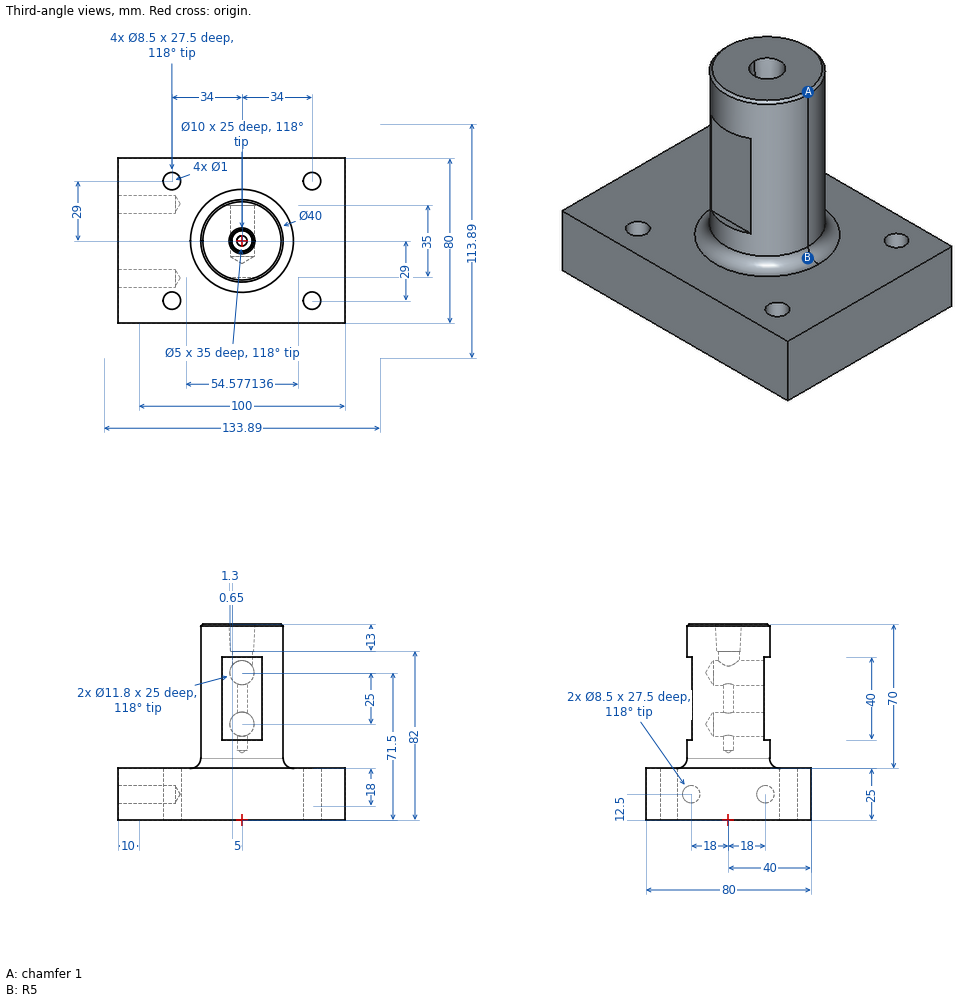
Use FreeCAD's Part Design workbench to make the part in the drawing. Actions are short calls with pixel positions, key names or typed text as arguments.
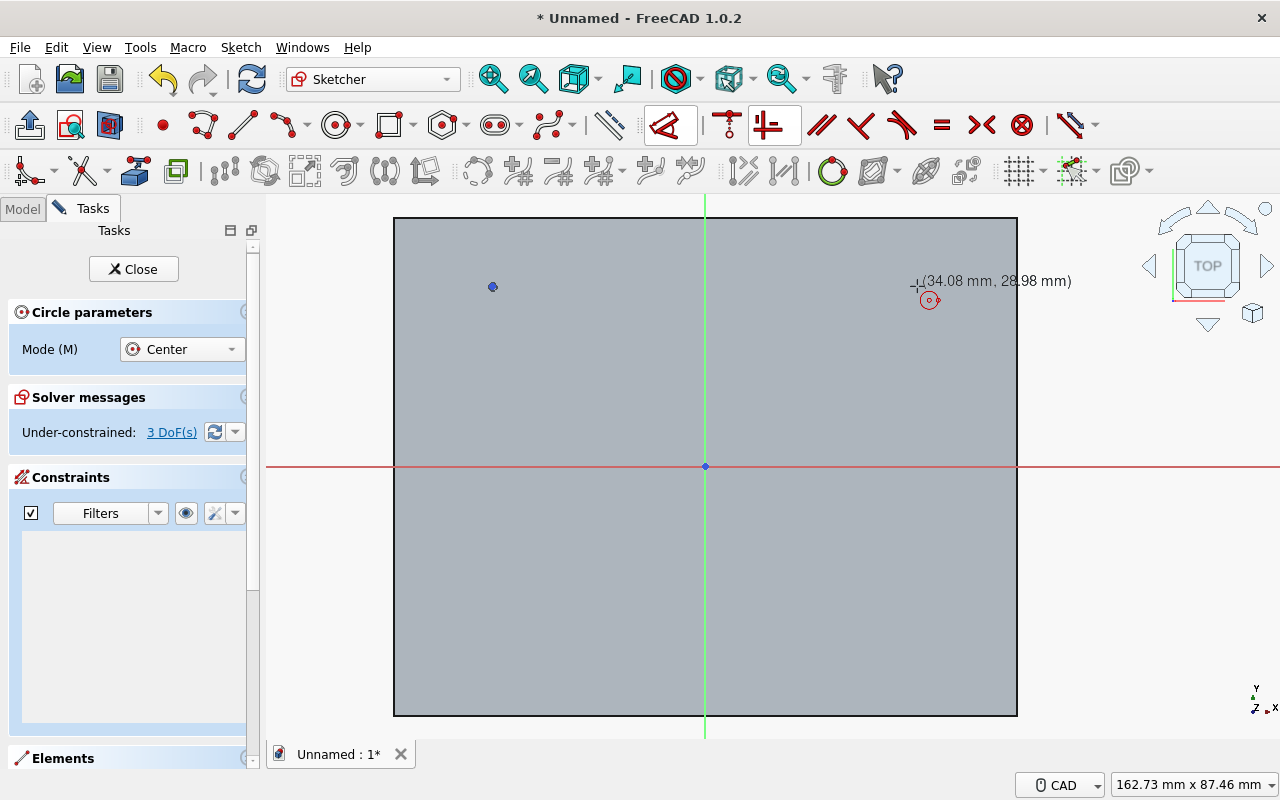
click(917, 286)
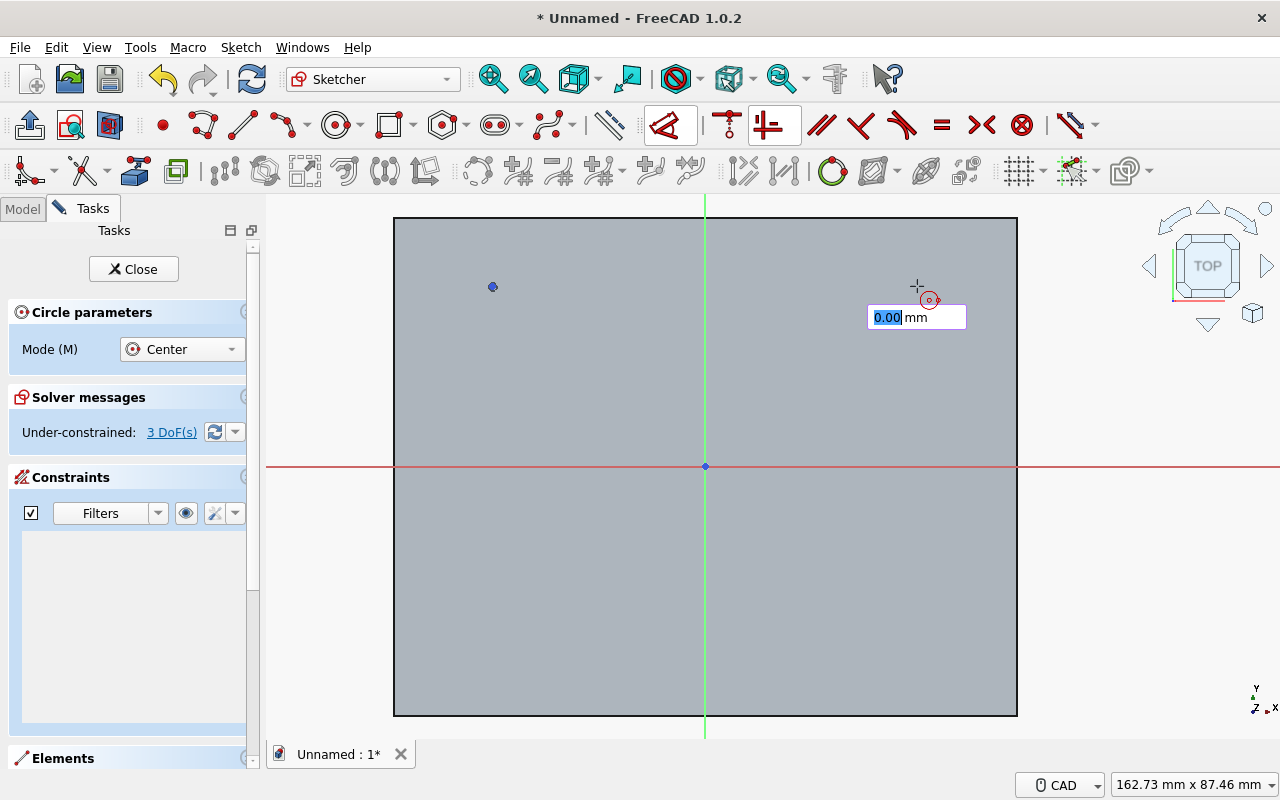
scroll(919, 284, up, 9)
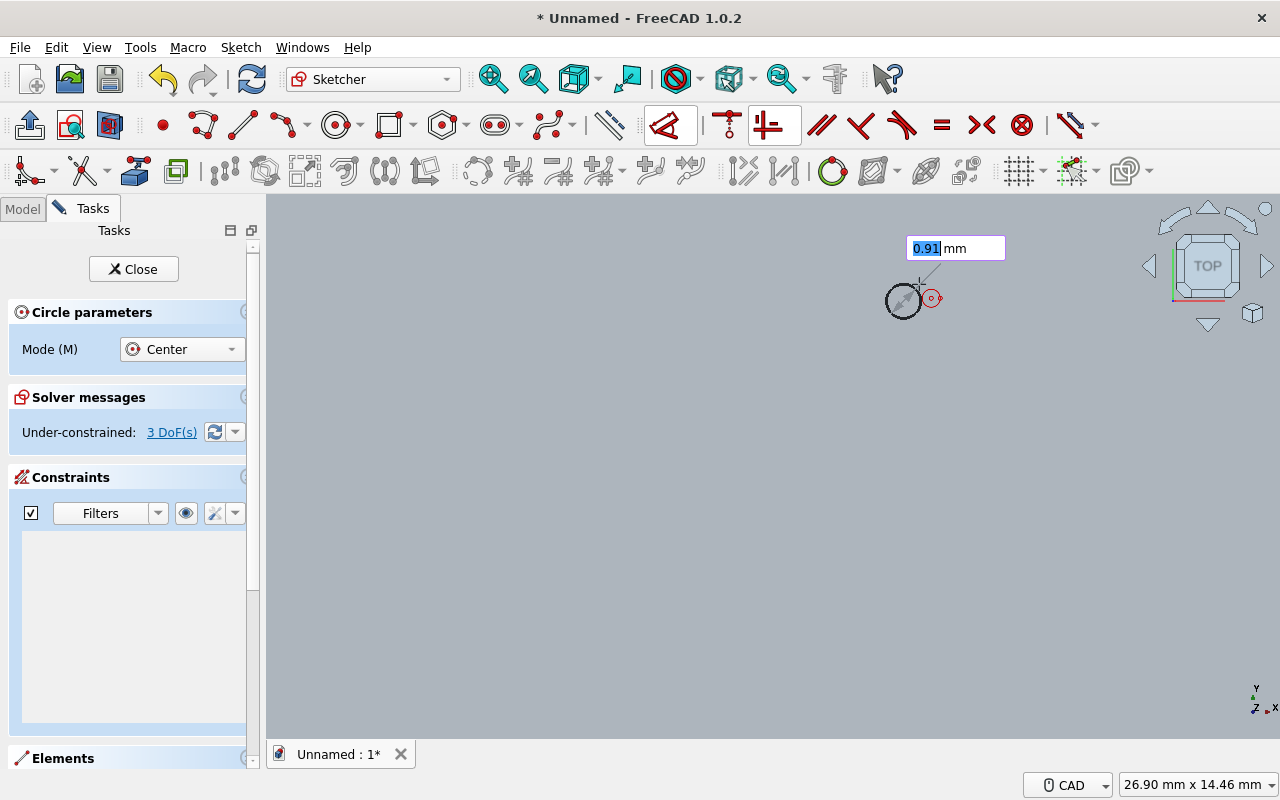
click(917, 283)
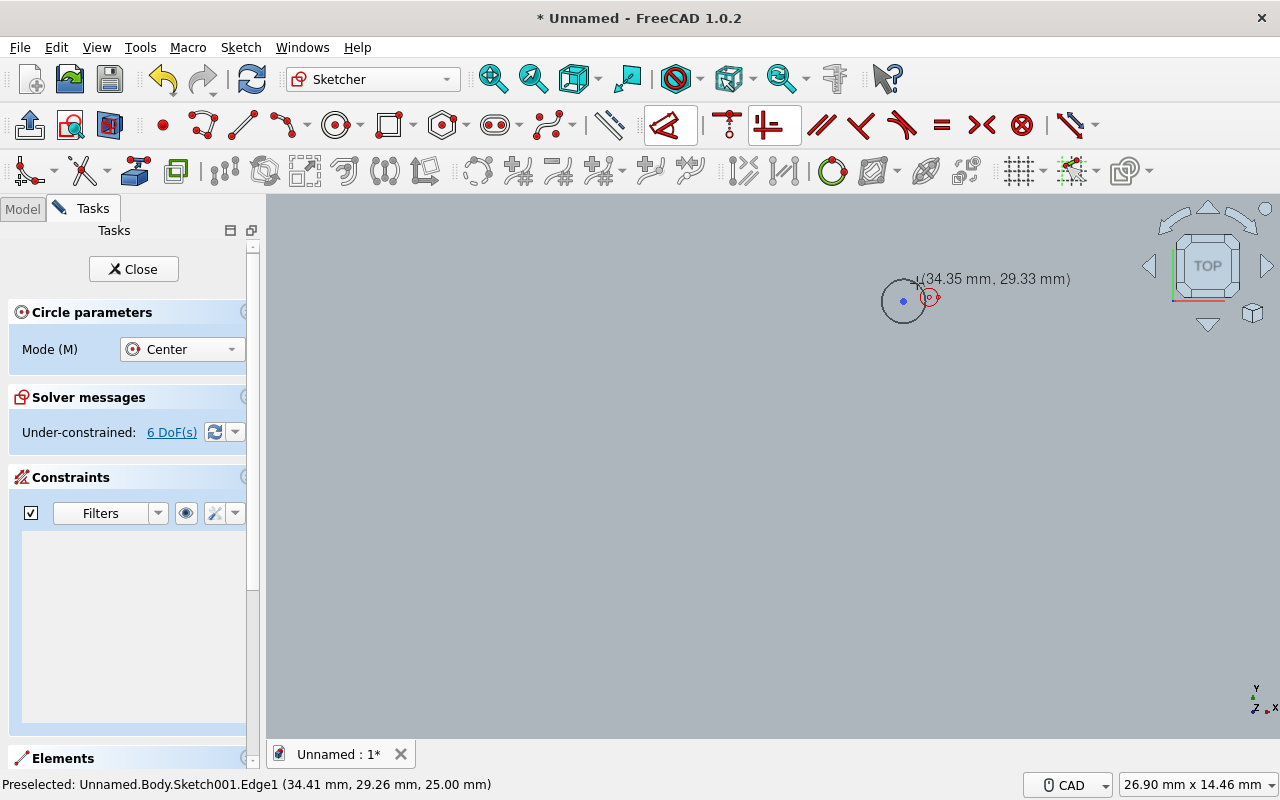
scroll(919, 284, down, 9)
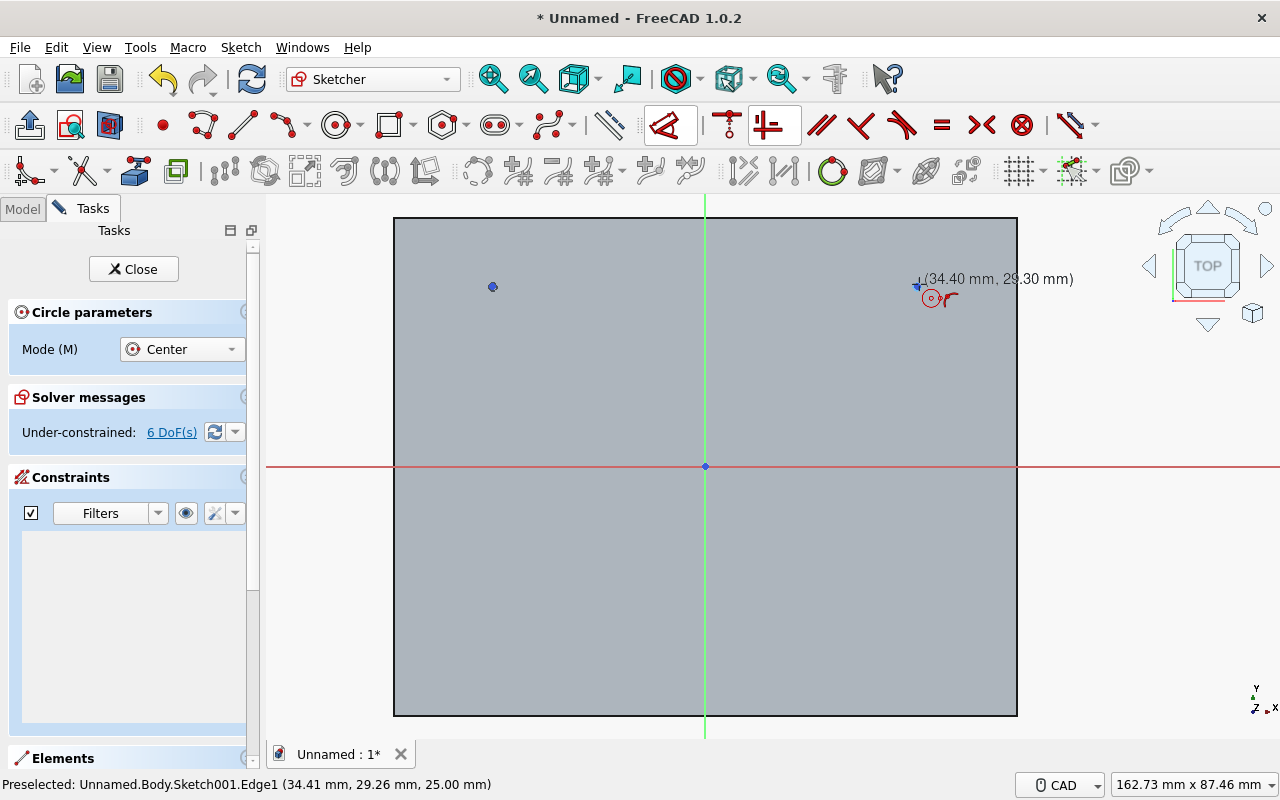
scroll(917, 648, up, 10)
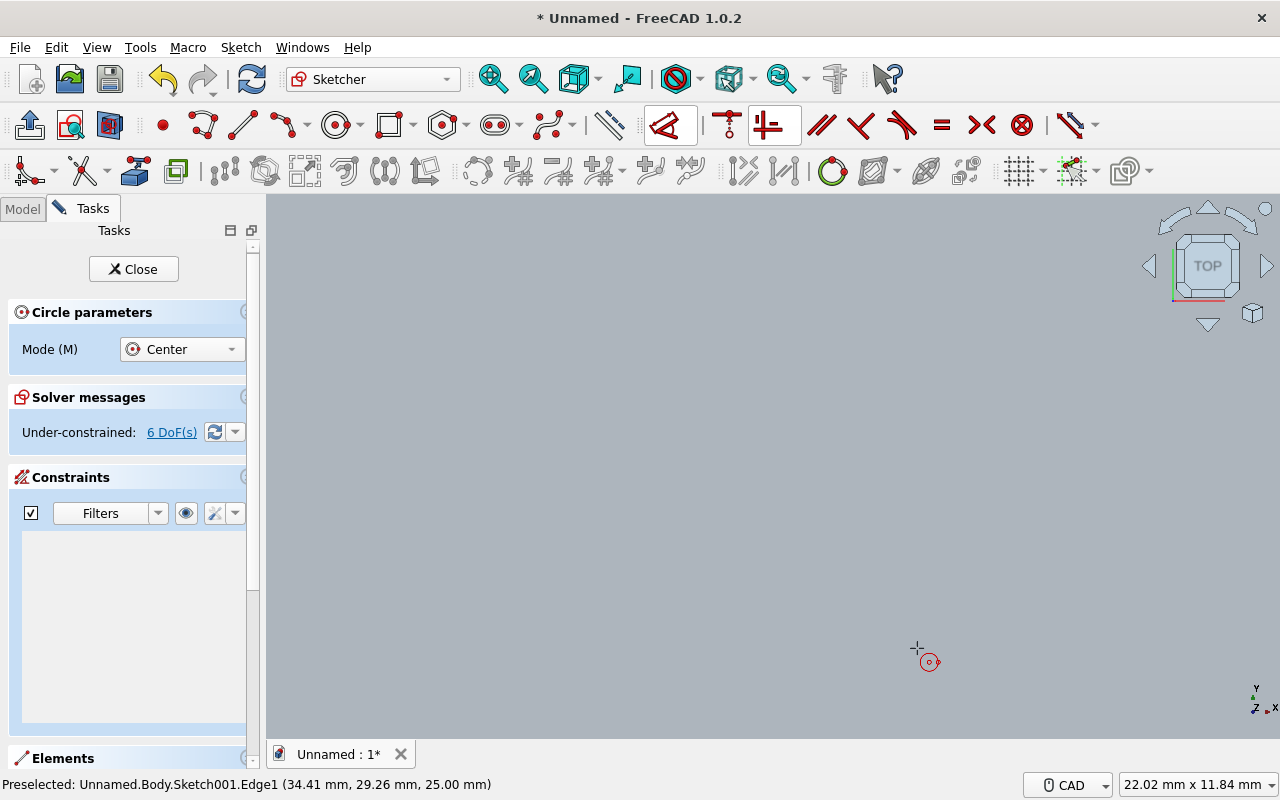
scroll(917, 648, down, 10)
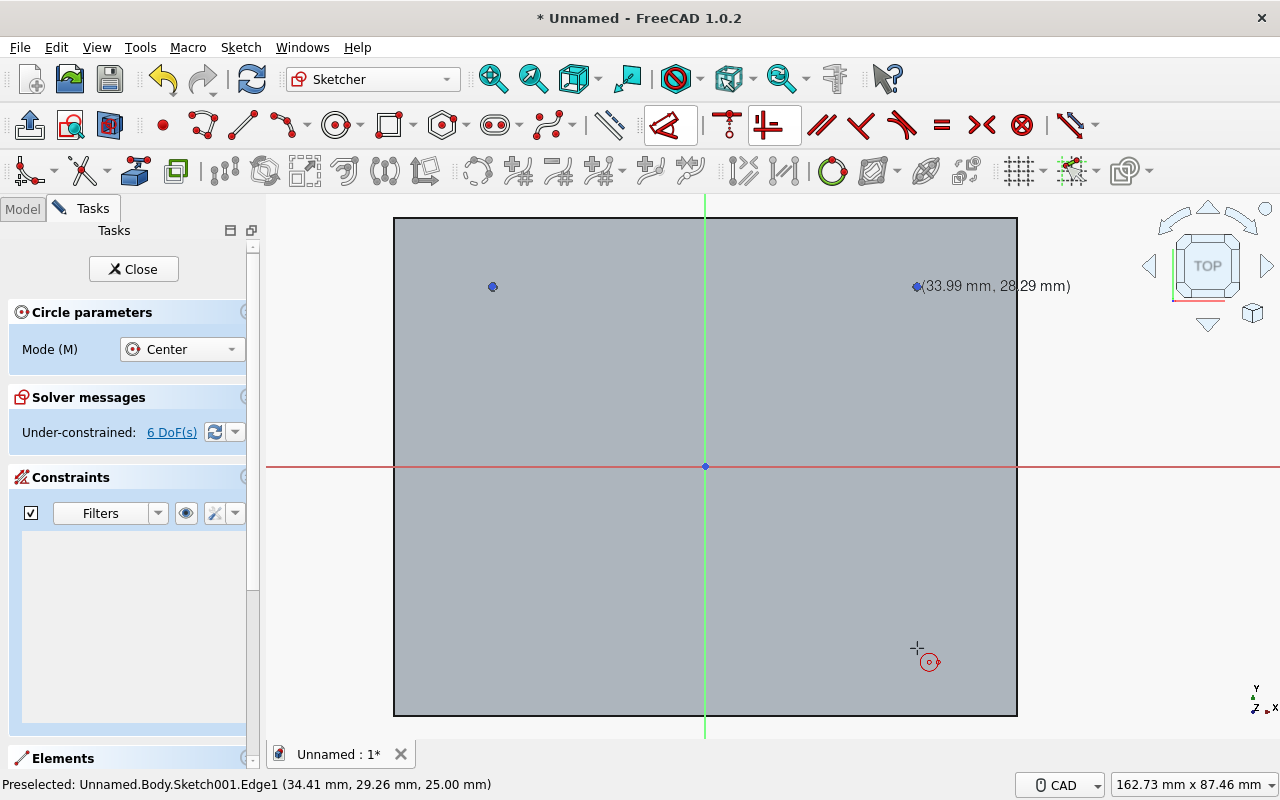
click(917, 648)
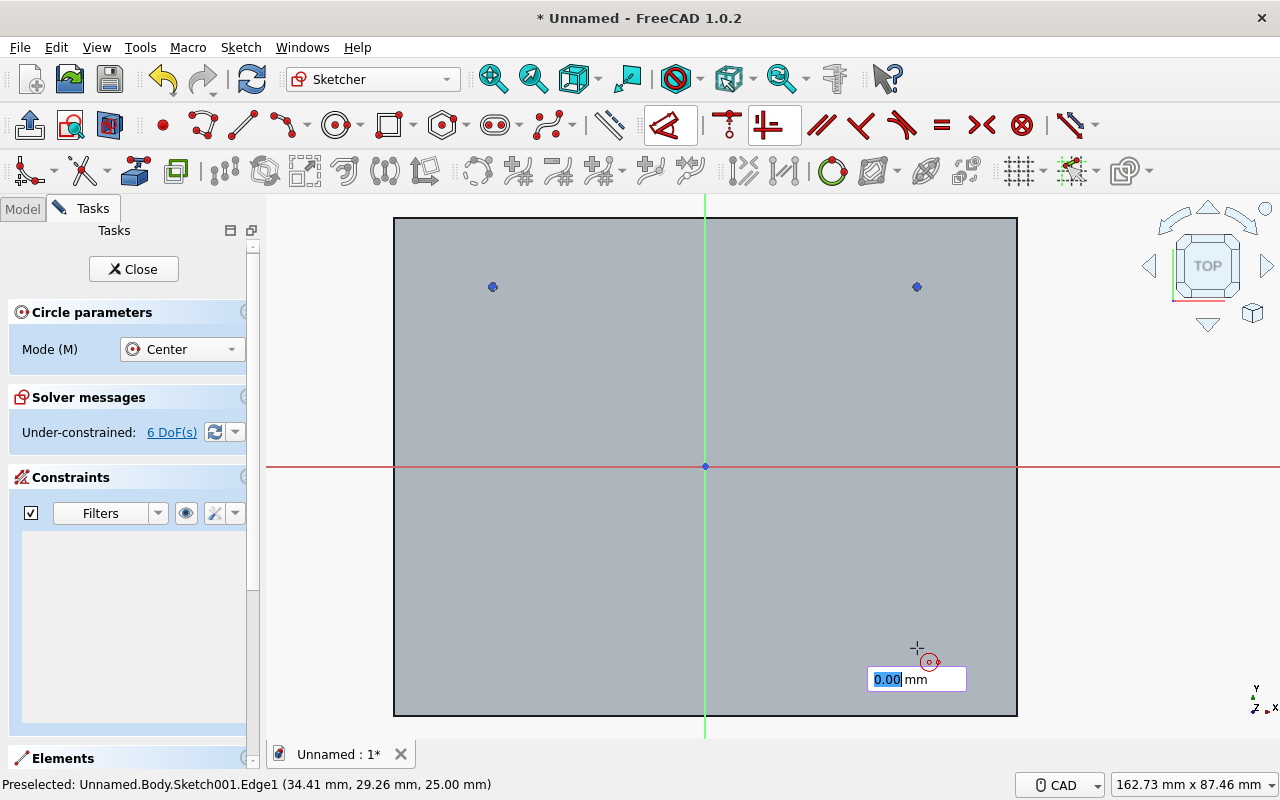
scroll(919, 645, up, 9)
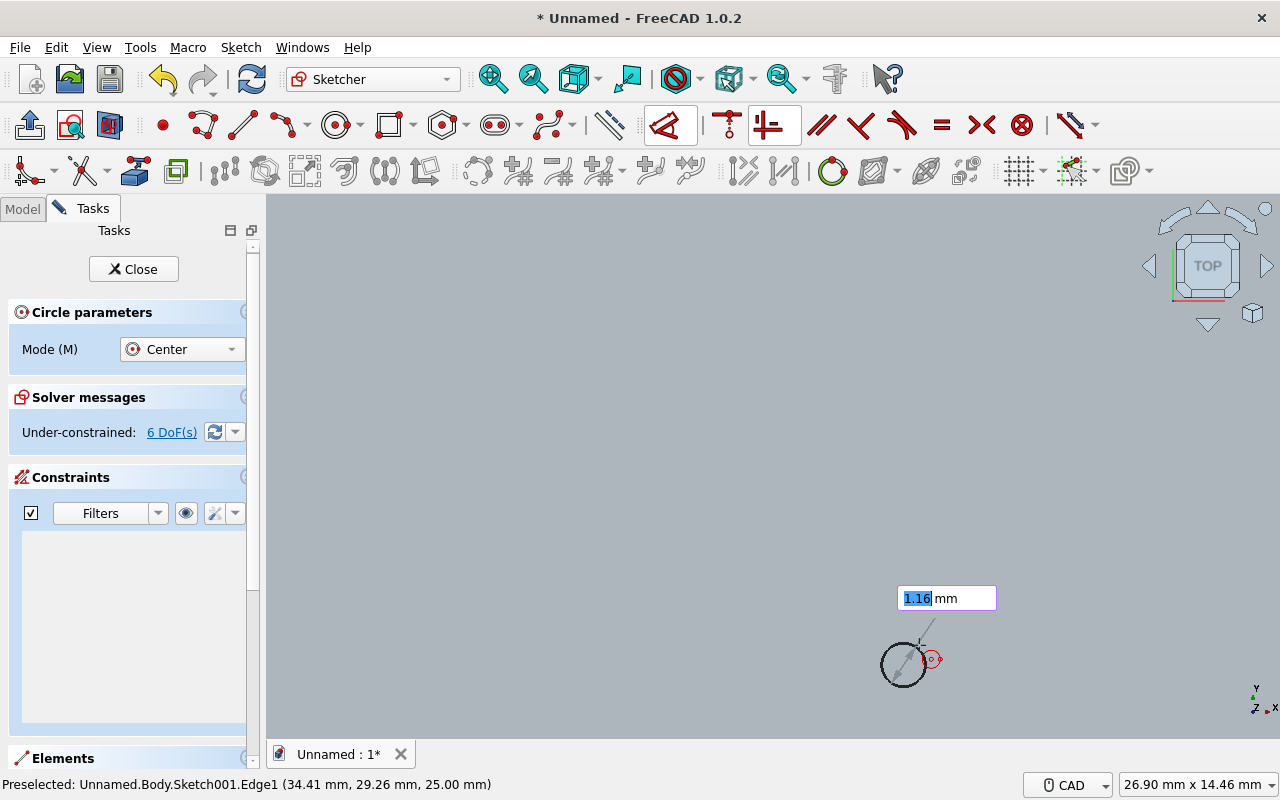
click(917, 643)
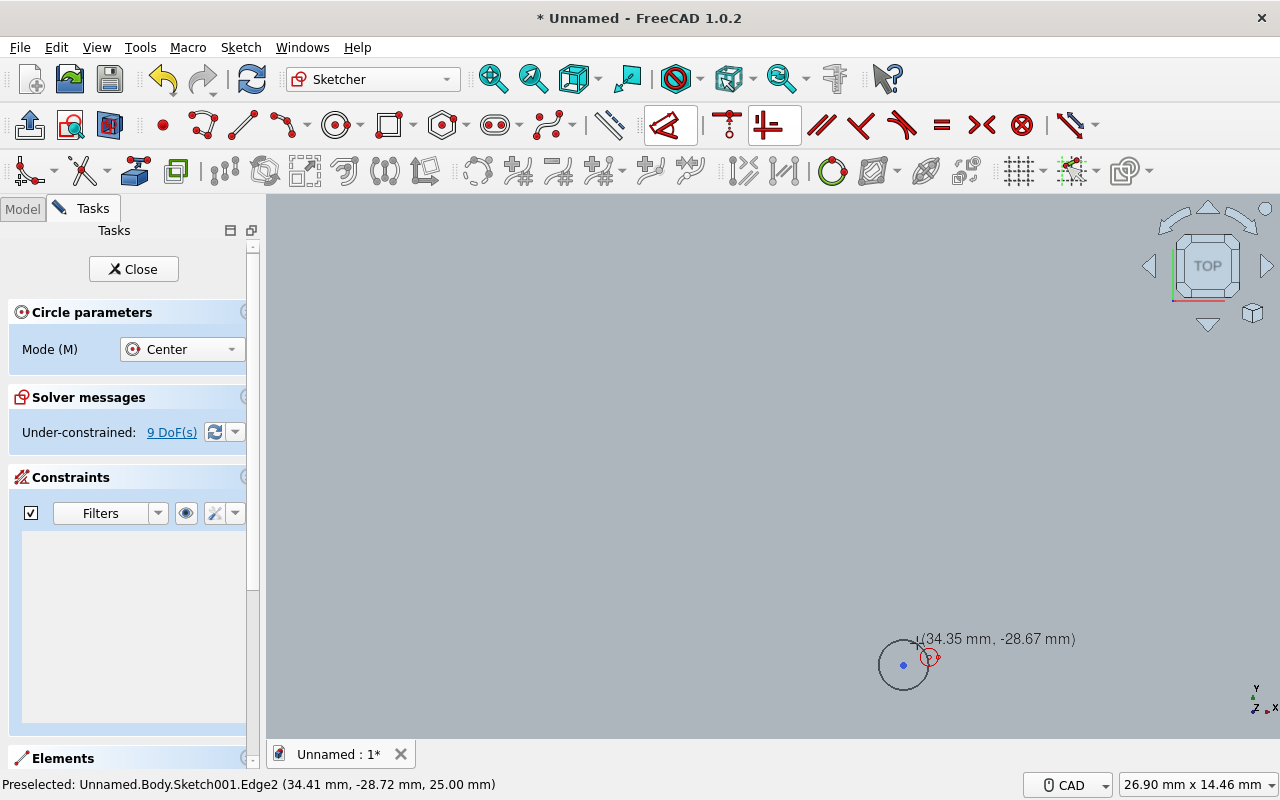
scroll(919, 645, down, 9)